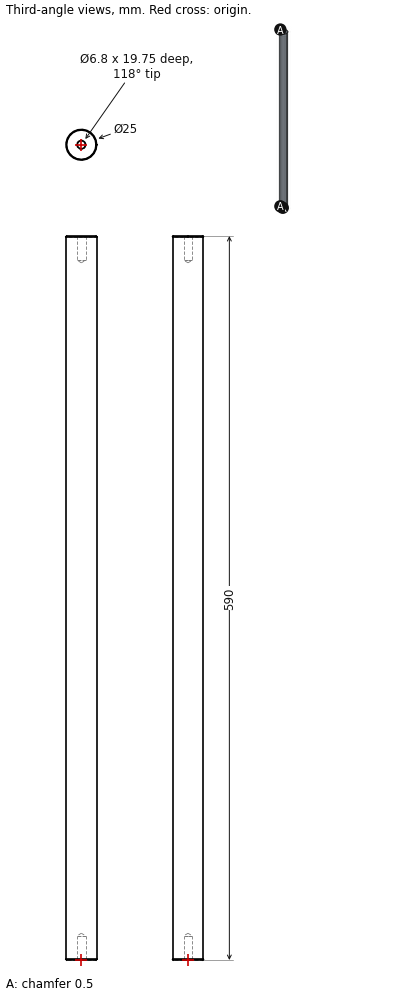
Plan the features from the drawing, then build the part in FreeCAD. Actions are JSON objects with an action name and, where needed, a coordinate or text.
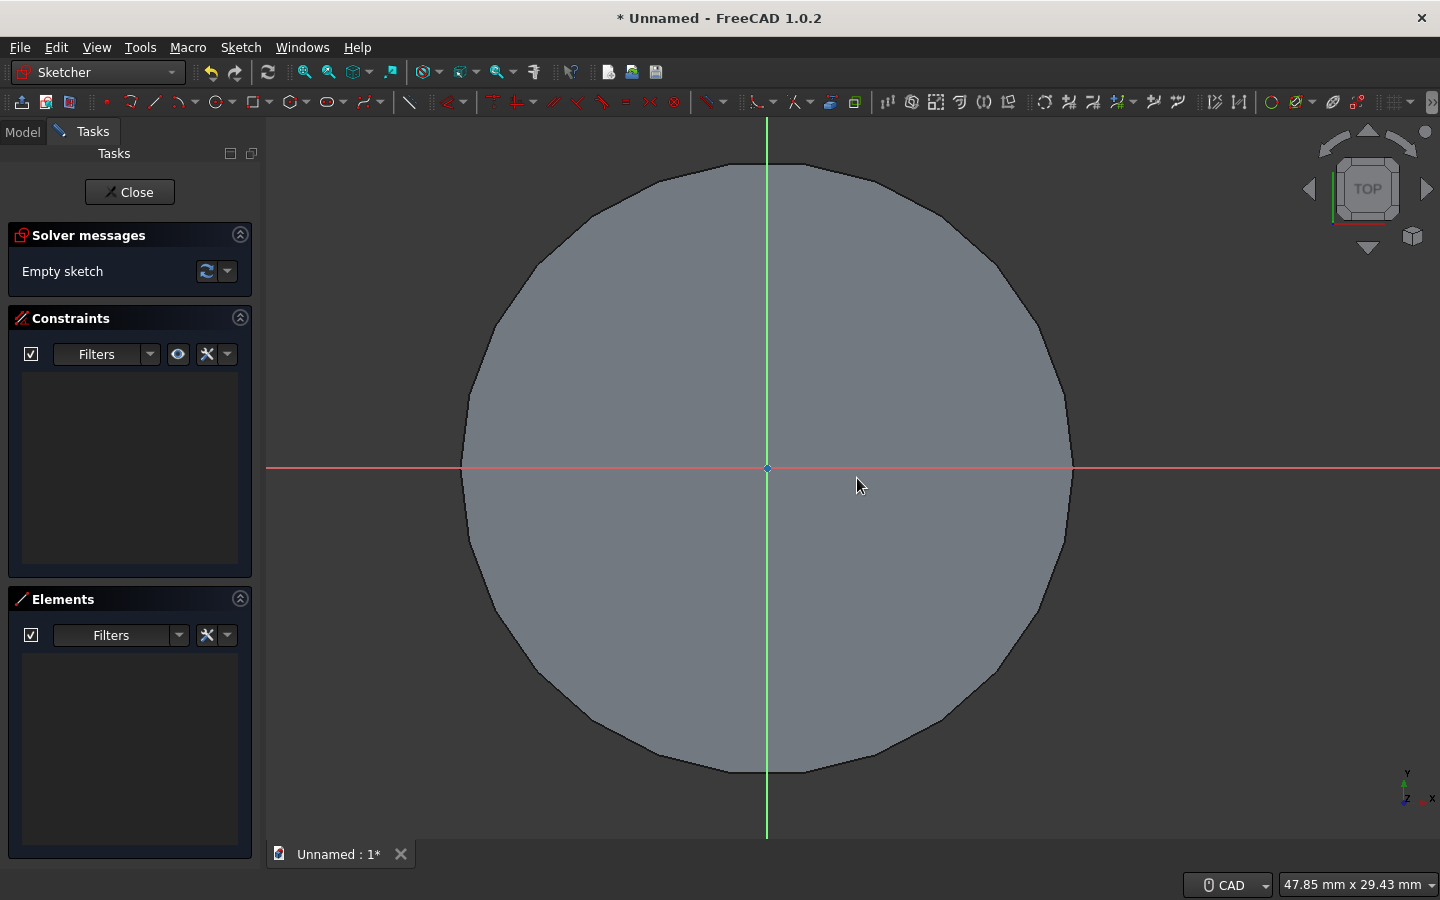
{"action": "scroll", "coordinate": [757, 463], "scroll_direction": "up", "scroll_amount": 5}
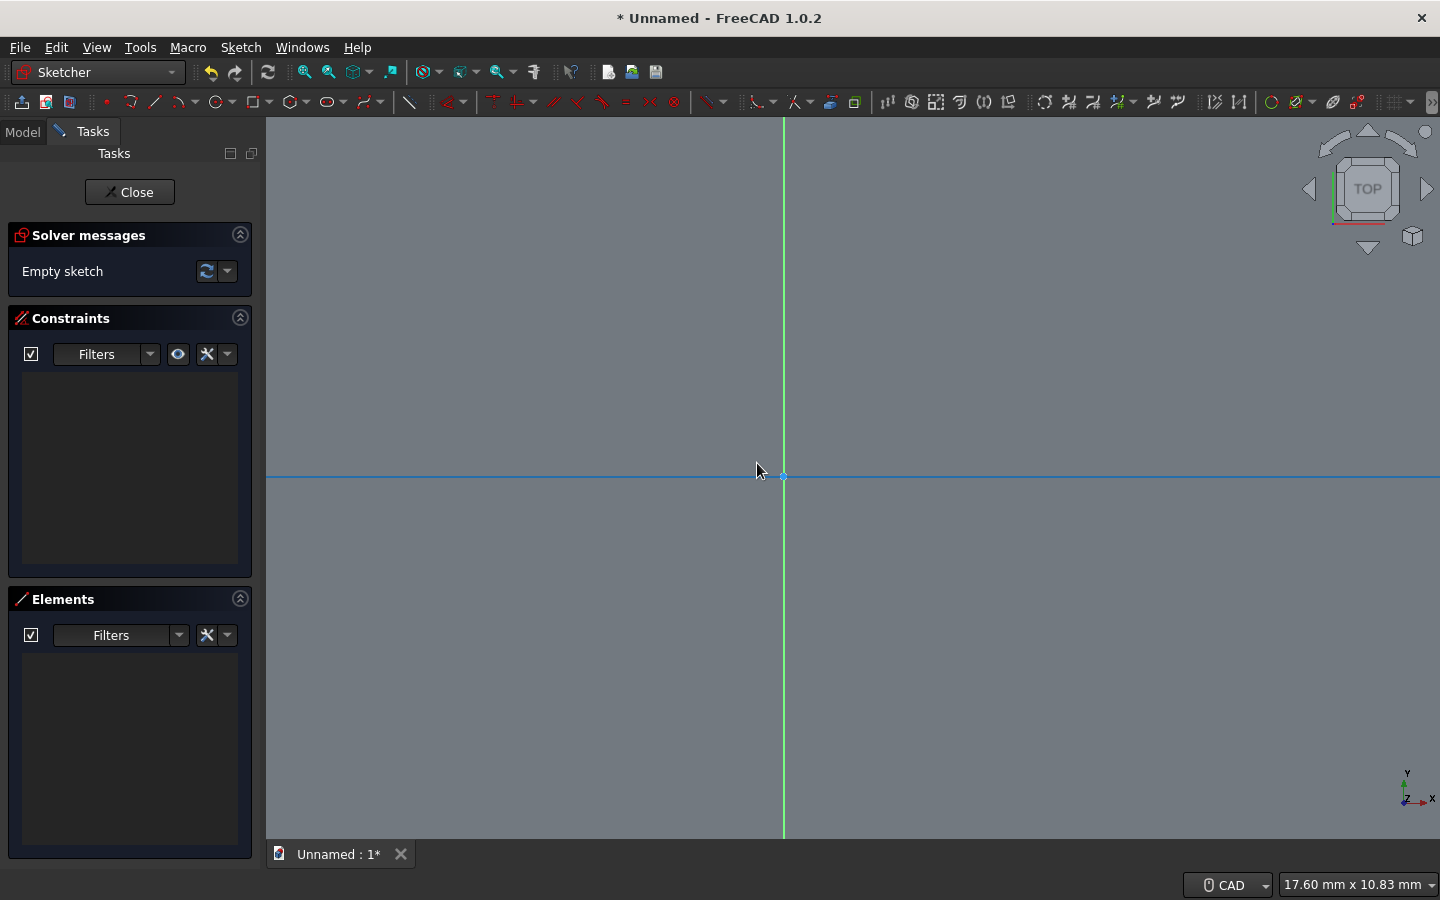
{"action": "key", "text": "g c"}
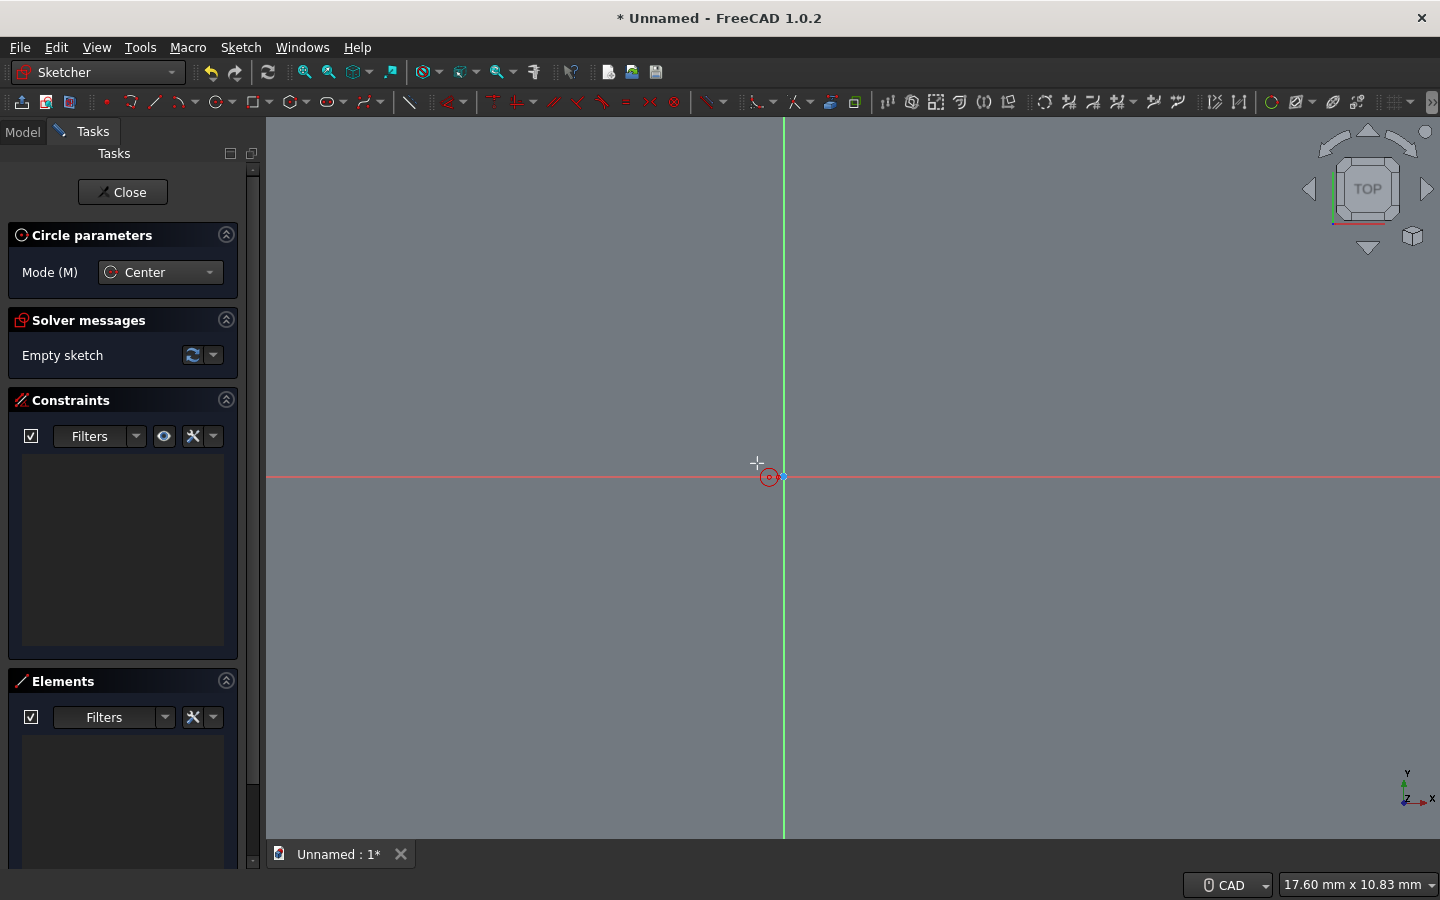
{"action": "left_click", "coordinate": [784, 477]}
{"action": "mouse_move", "coordinate": [944, 317]}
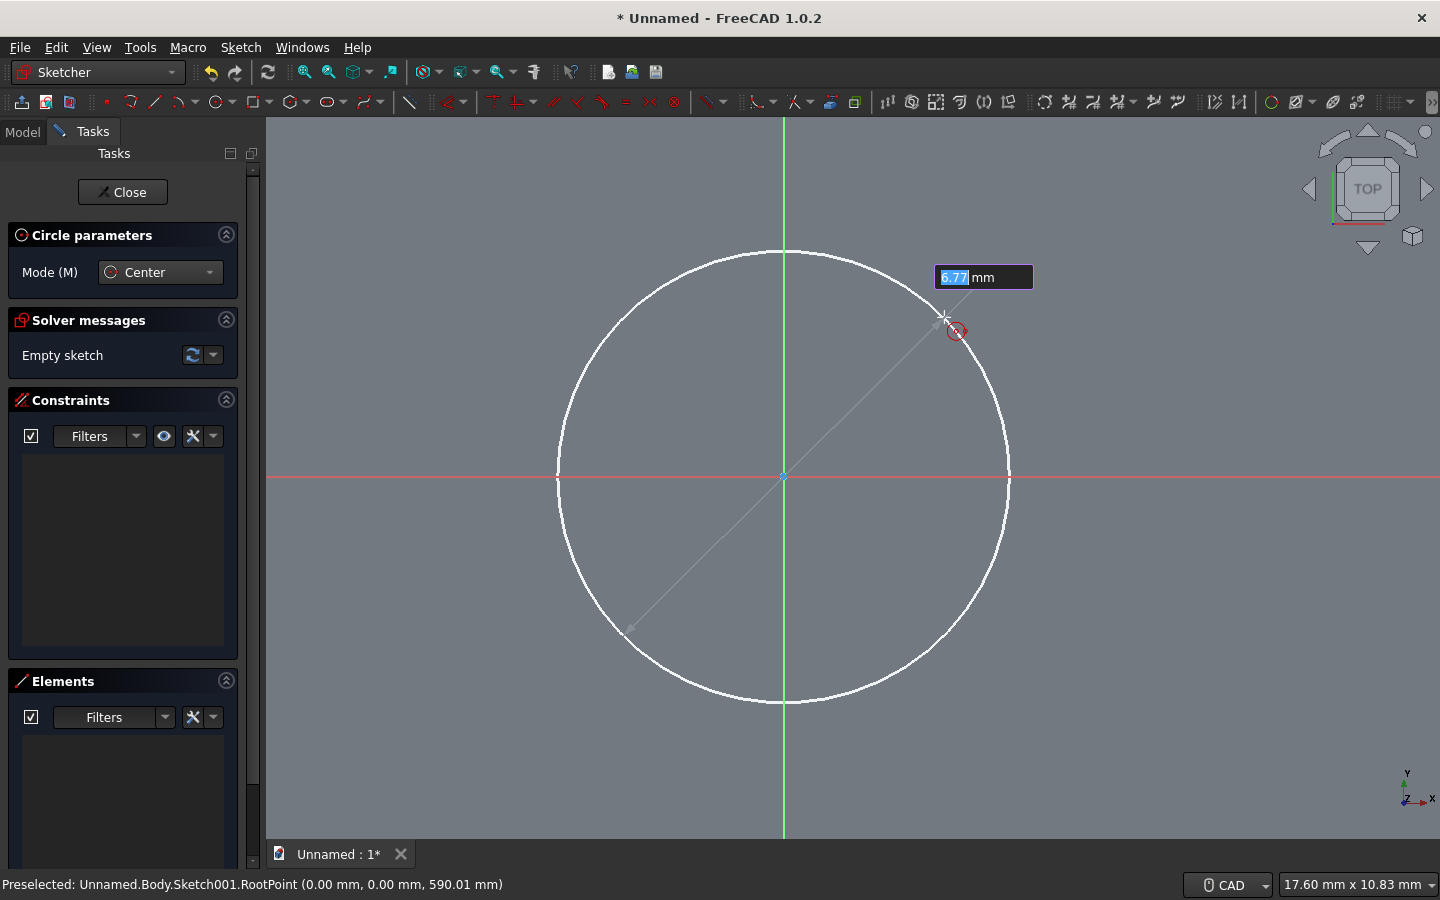
{"action": "type", "text": "6.8"}
{"action": "key", "text": "Return"}
{"action": "key", "text": "Escape"}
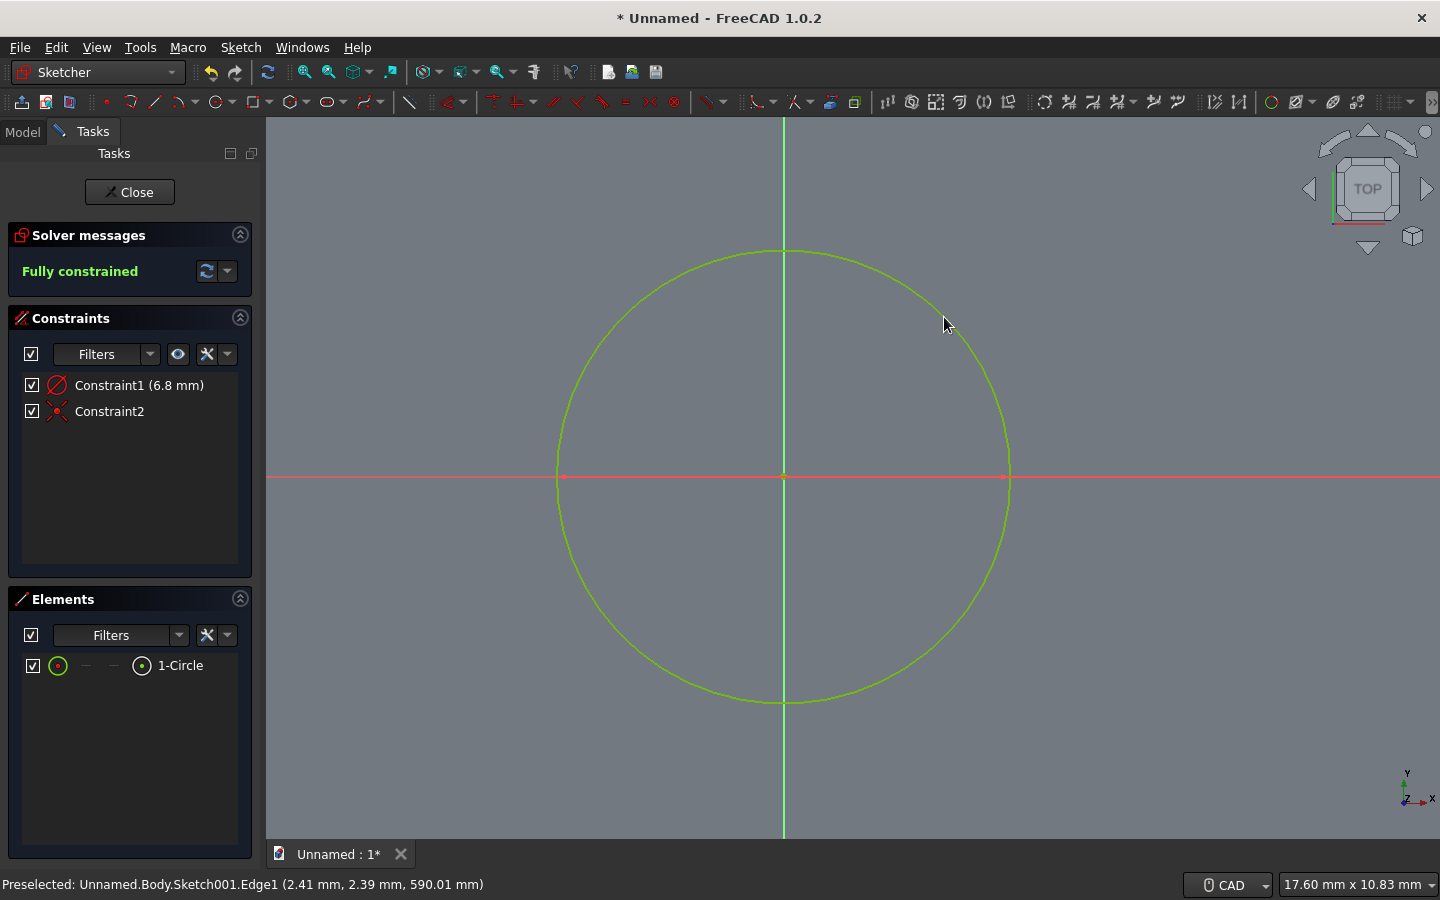
{"action": "left_click", "coordinate": [130, 192]}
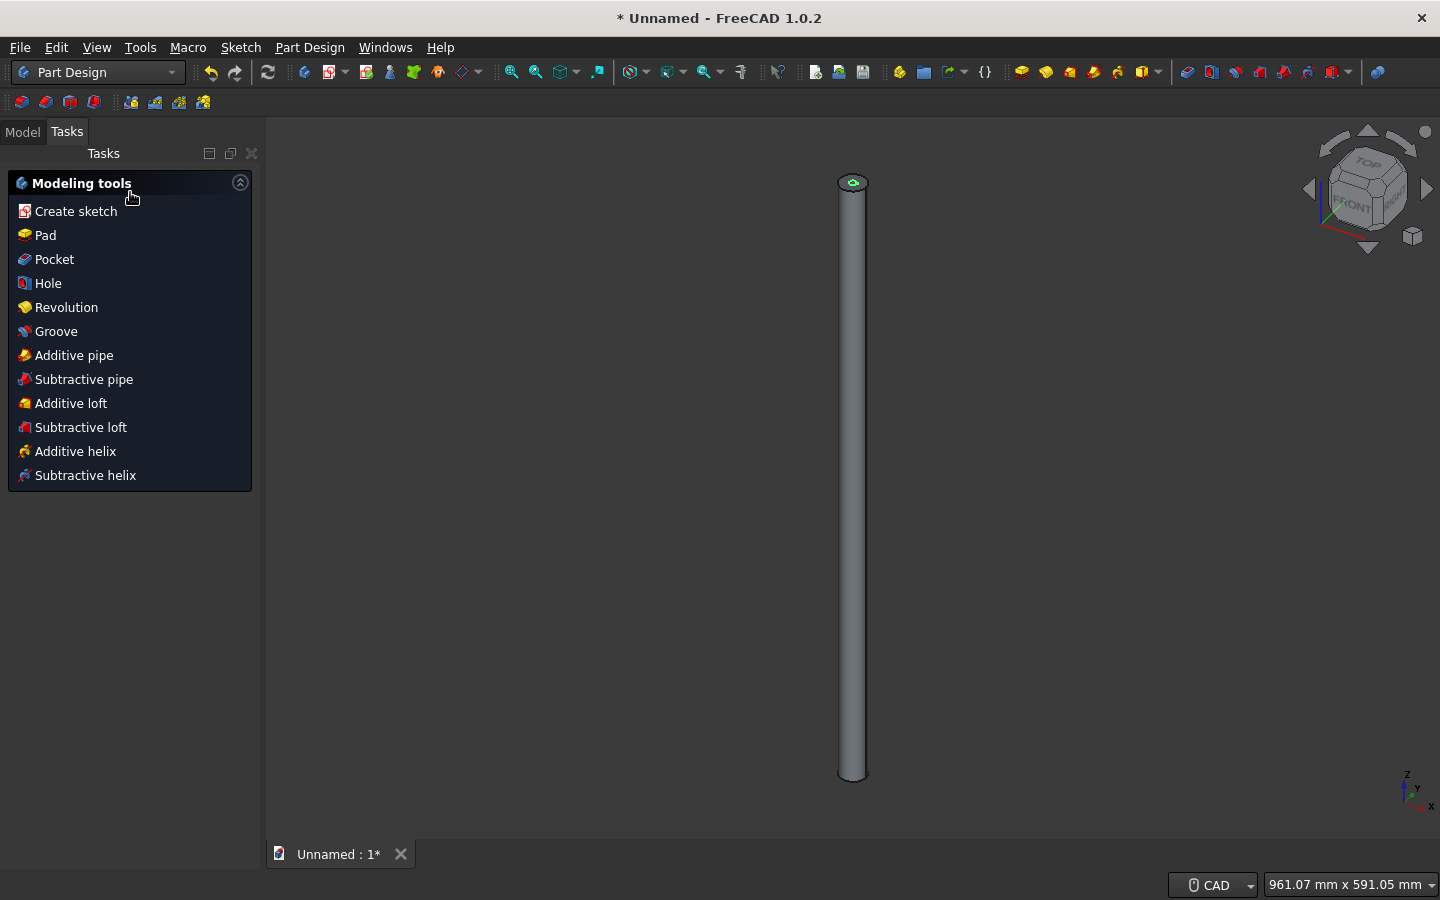
{"action": "left_click", "coordinate": [1212, 72]}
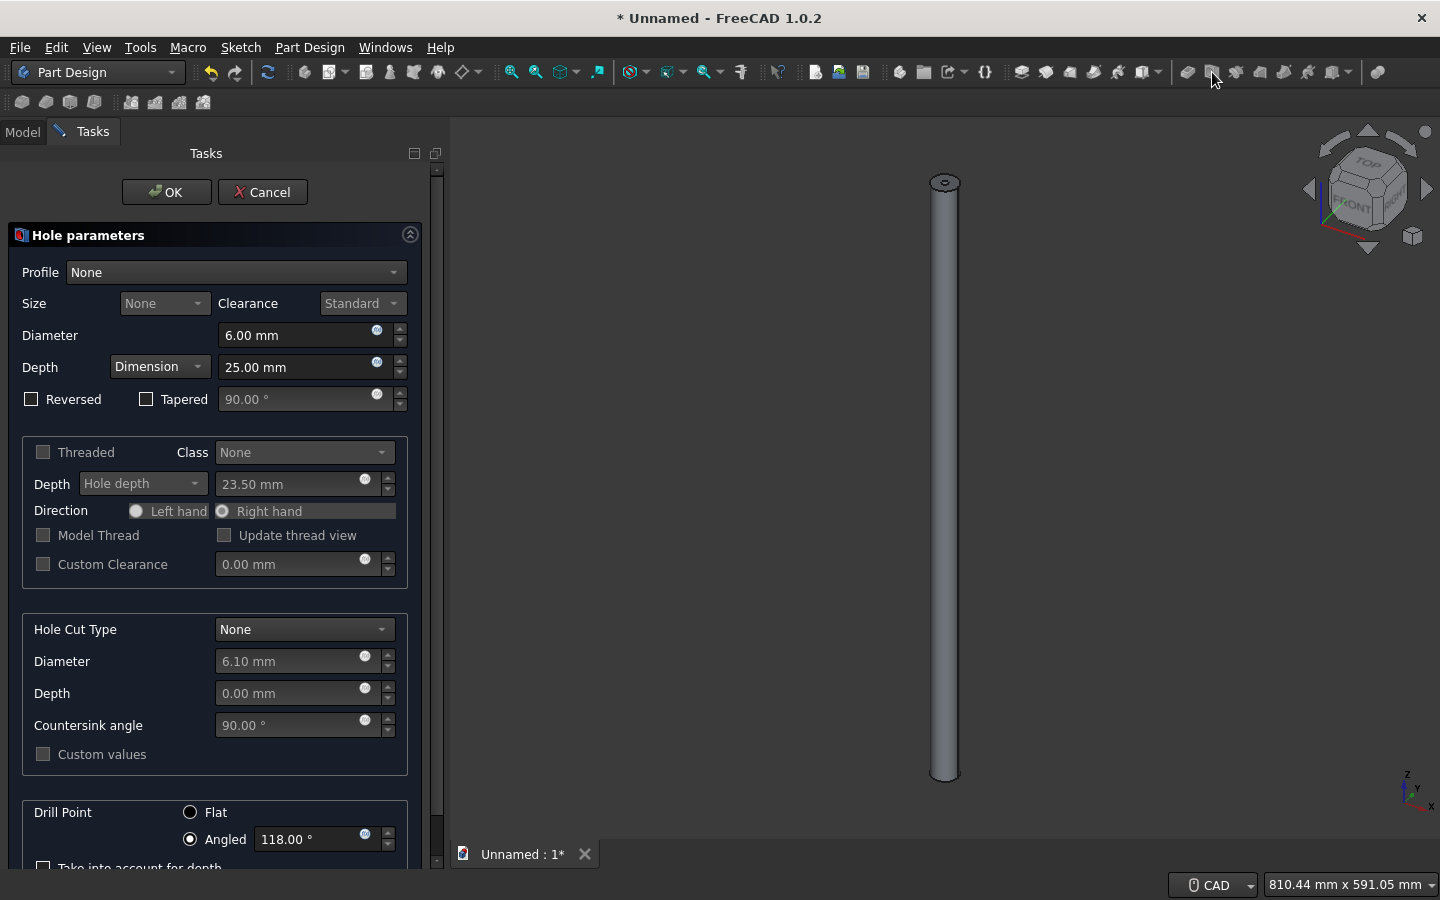
{"action": "triple_click", "coordinate": [305, 335]}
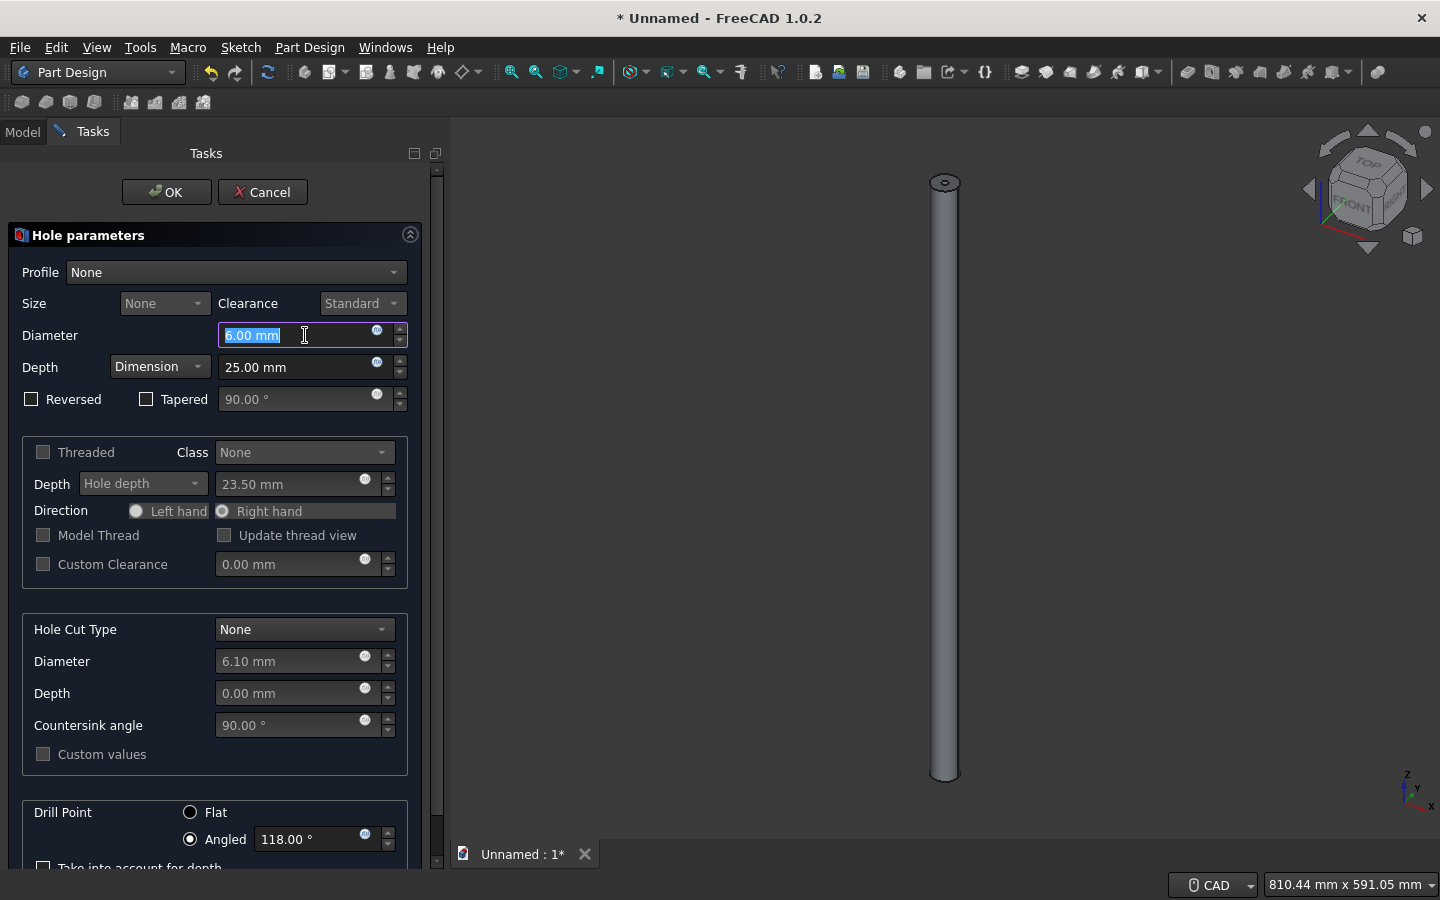
{"action": "type", "text": "6.8"}
{"action": "key", "text": "Tab"}